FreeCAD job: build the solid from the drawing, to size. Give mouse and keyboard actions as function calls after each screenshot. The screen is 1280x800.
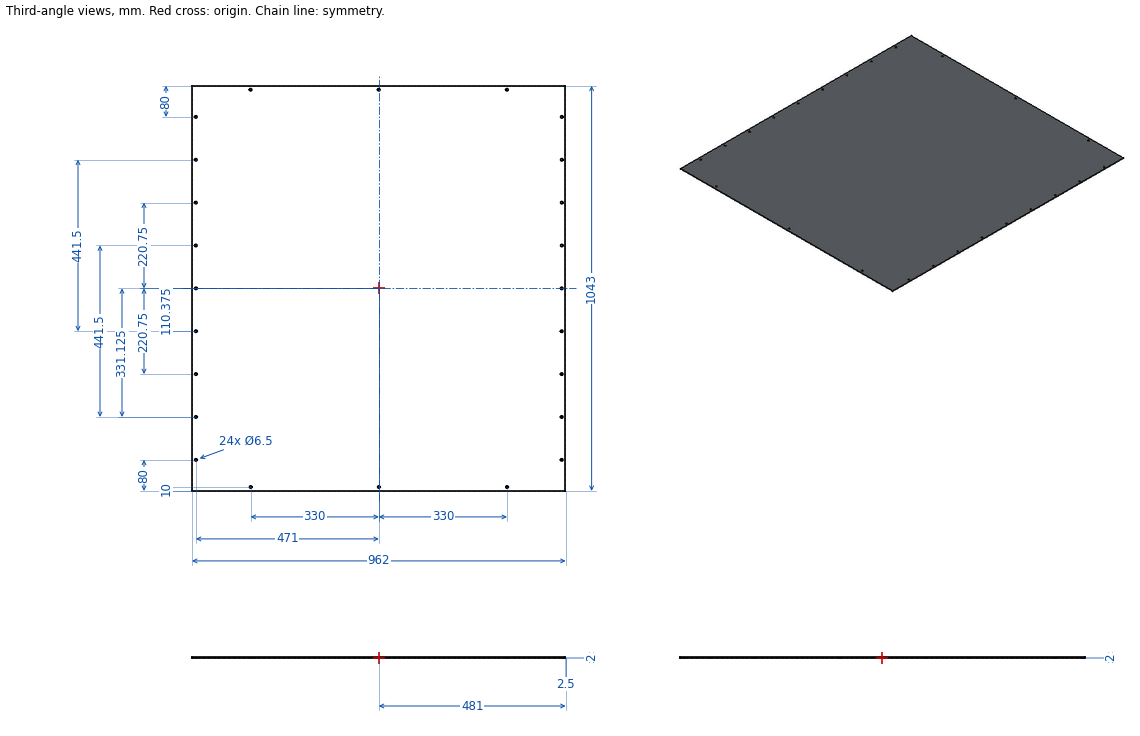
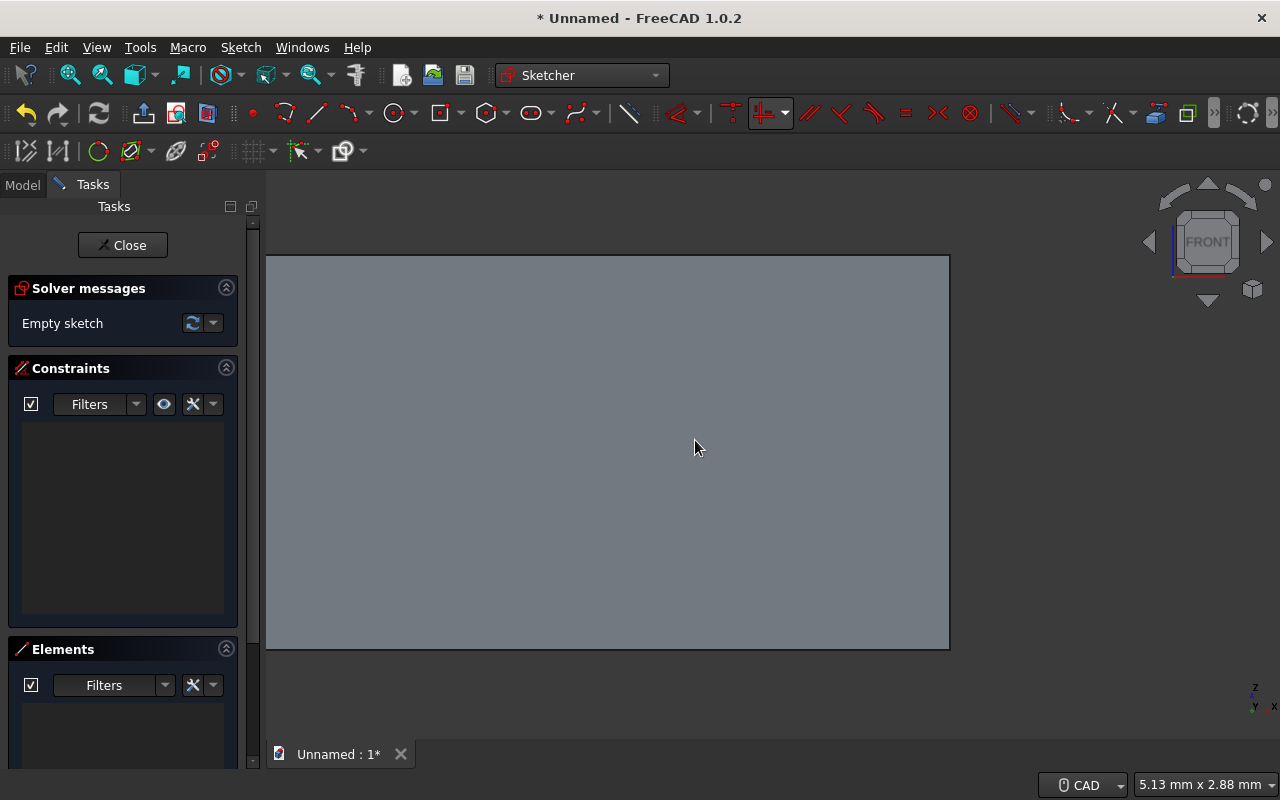
key(g)
key(r)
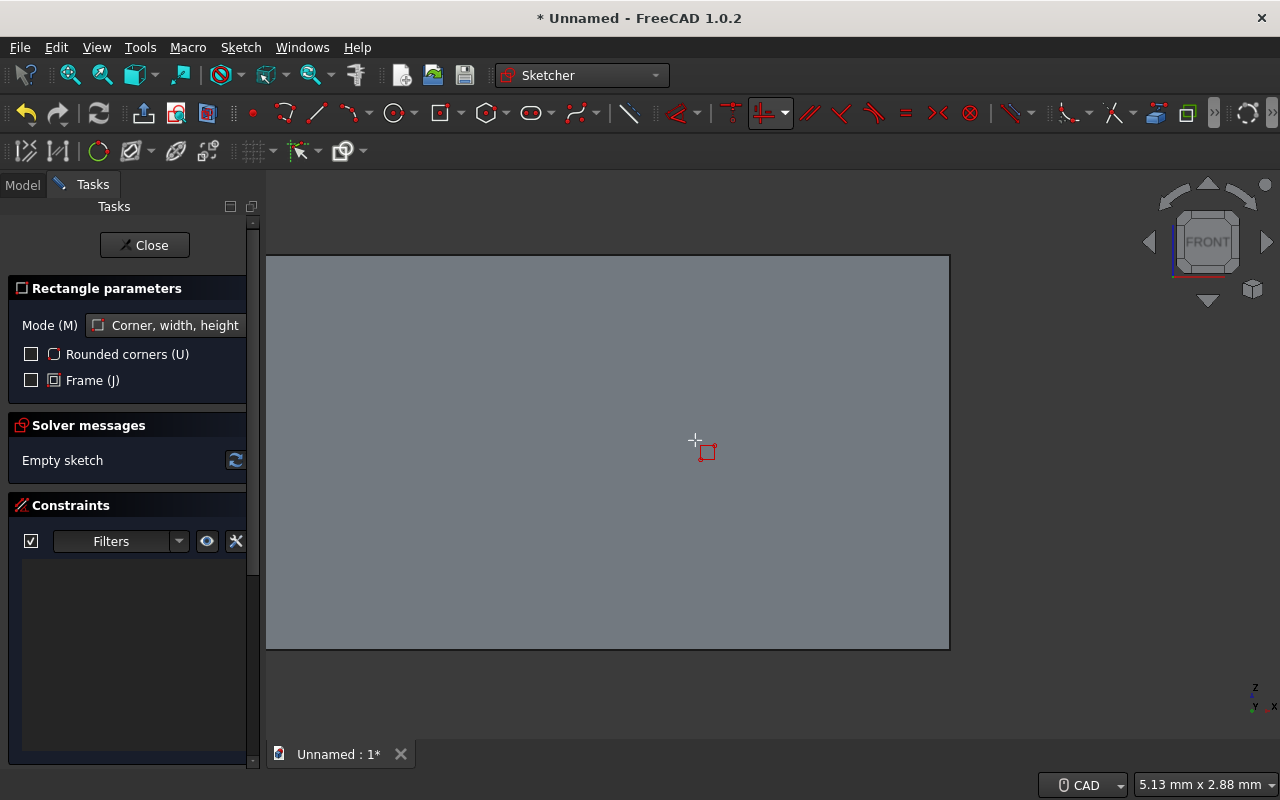
click(456, 255)
click(950, 650)
key(Escape)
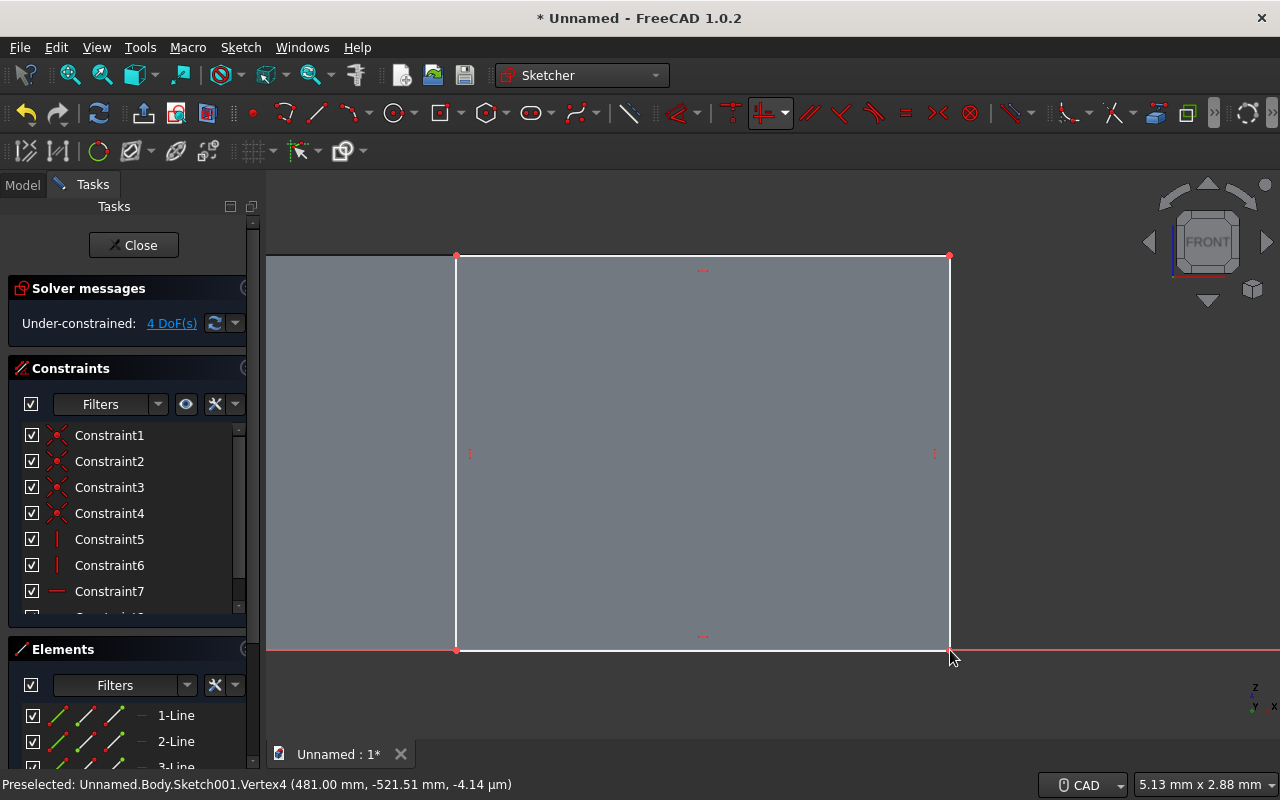
click(456, 651)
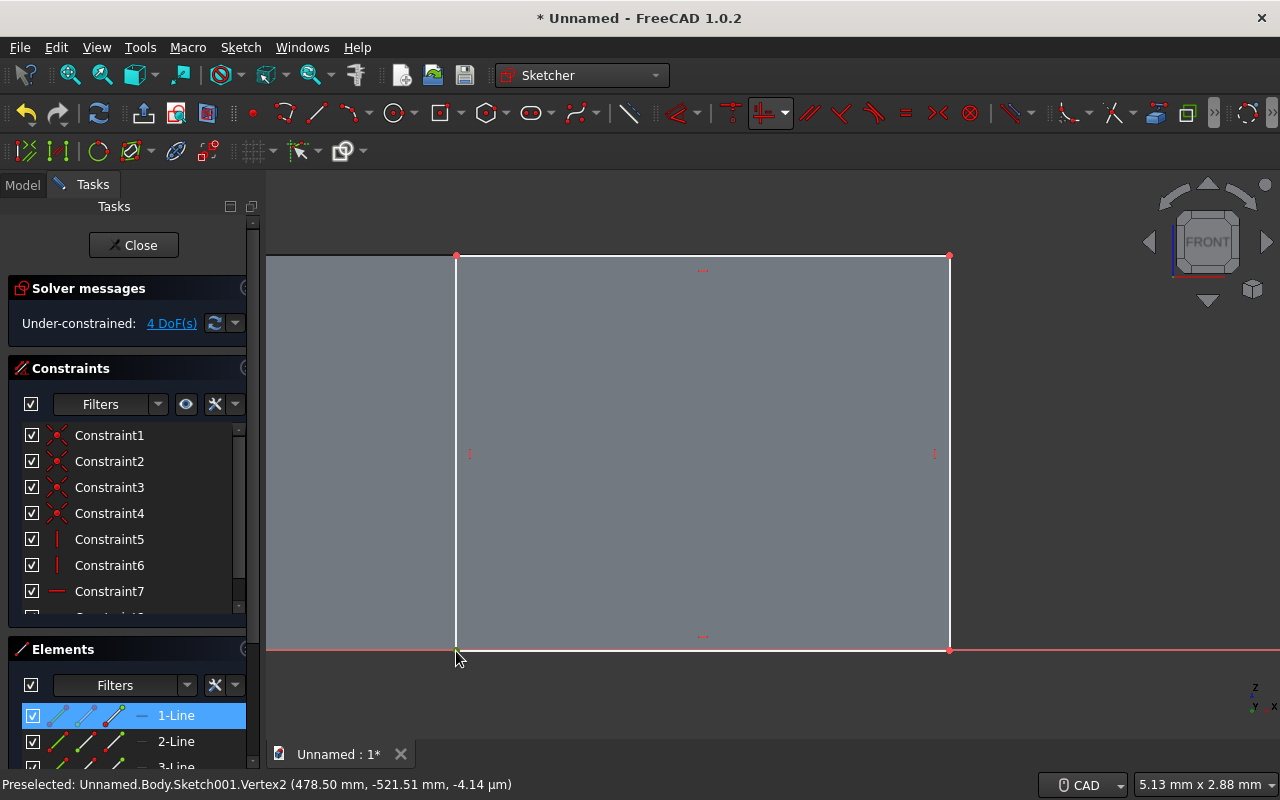
click(353, 650)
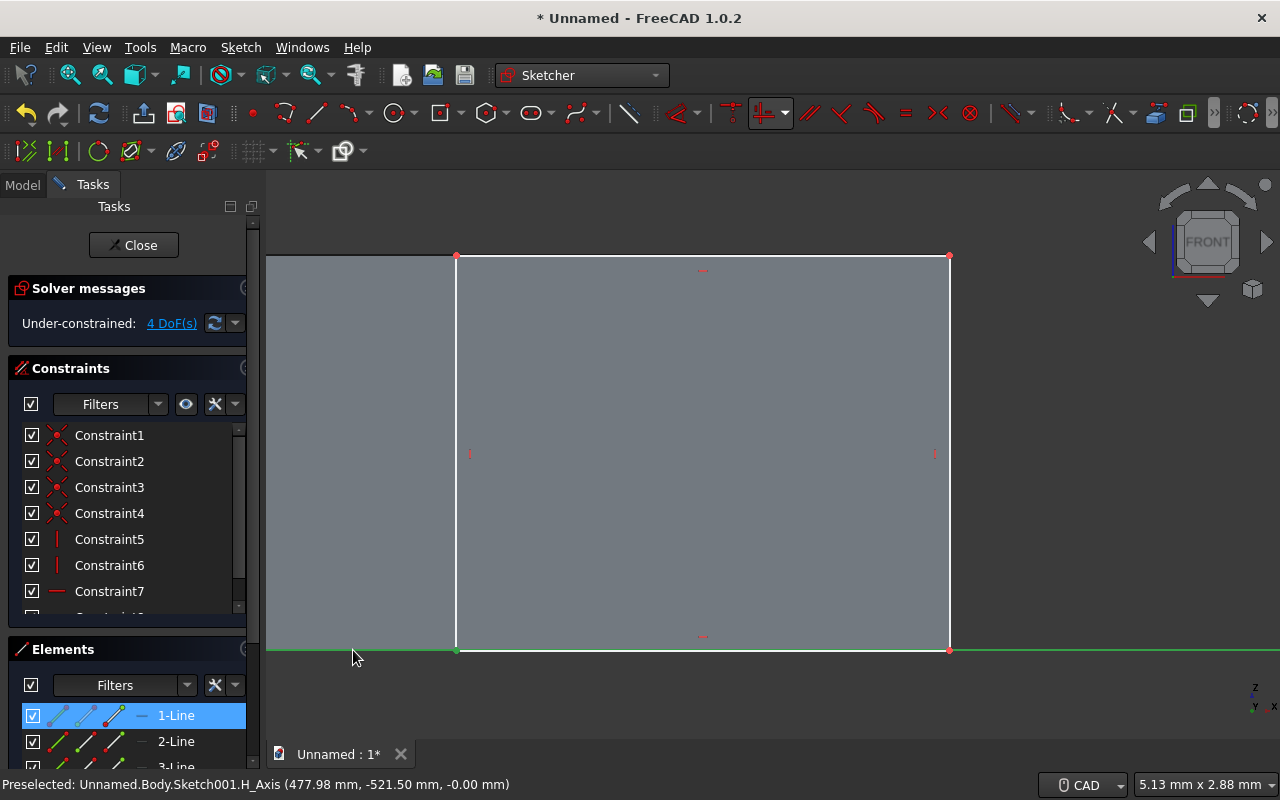
click(732, 114)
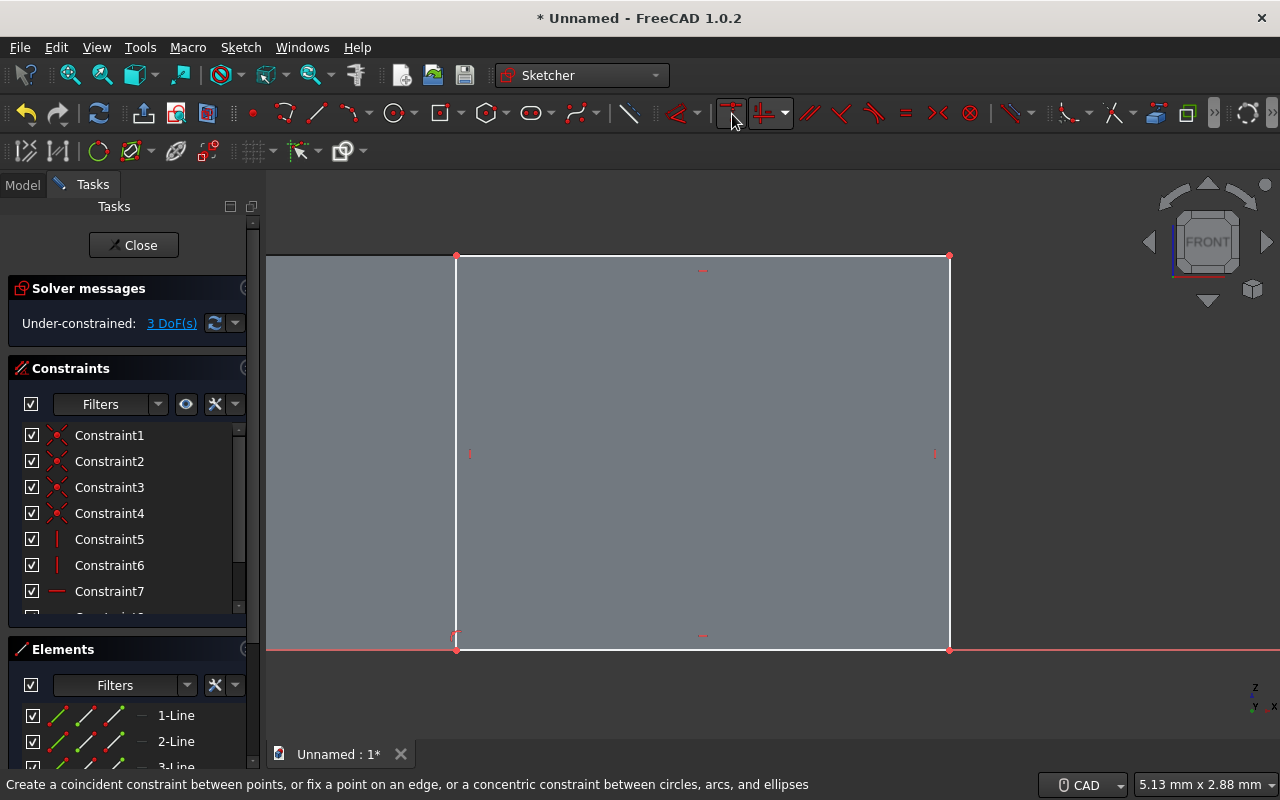
click(676, 114)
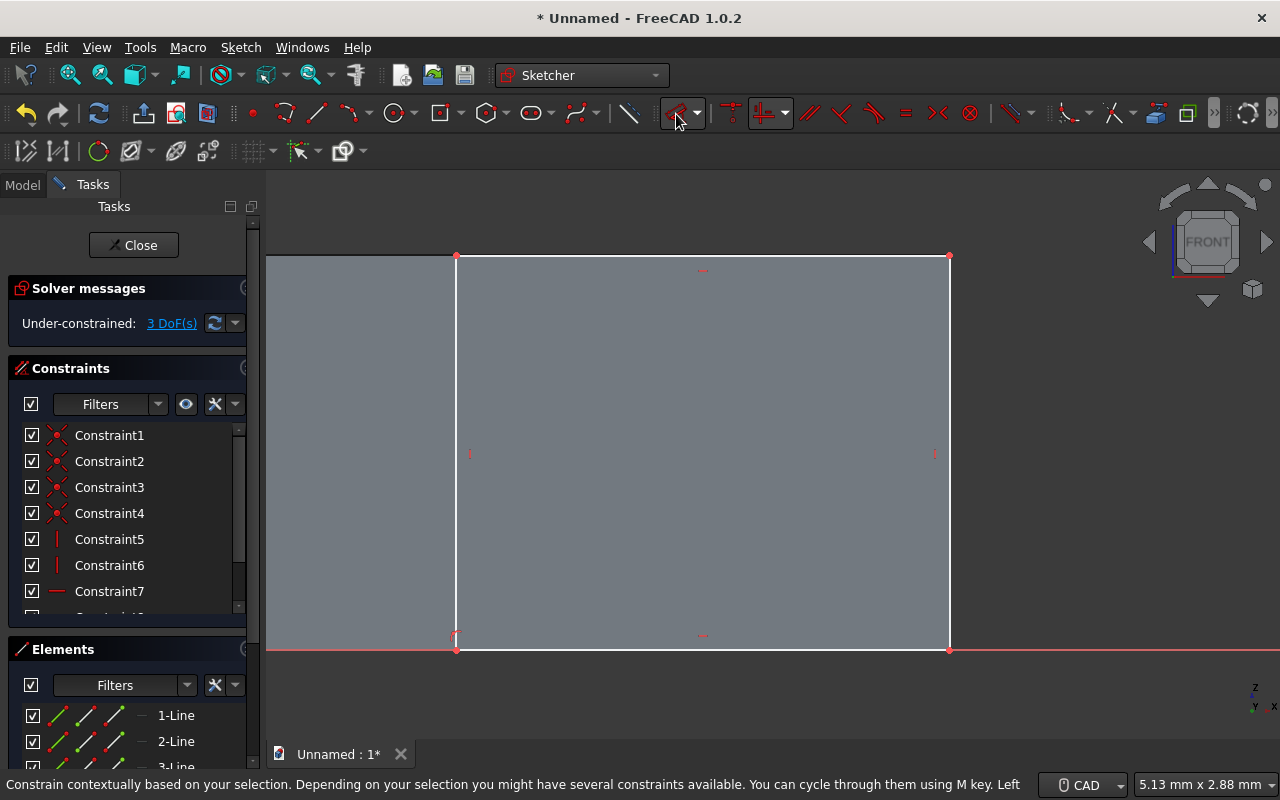
click(456, 374)
click(422, 453)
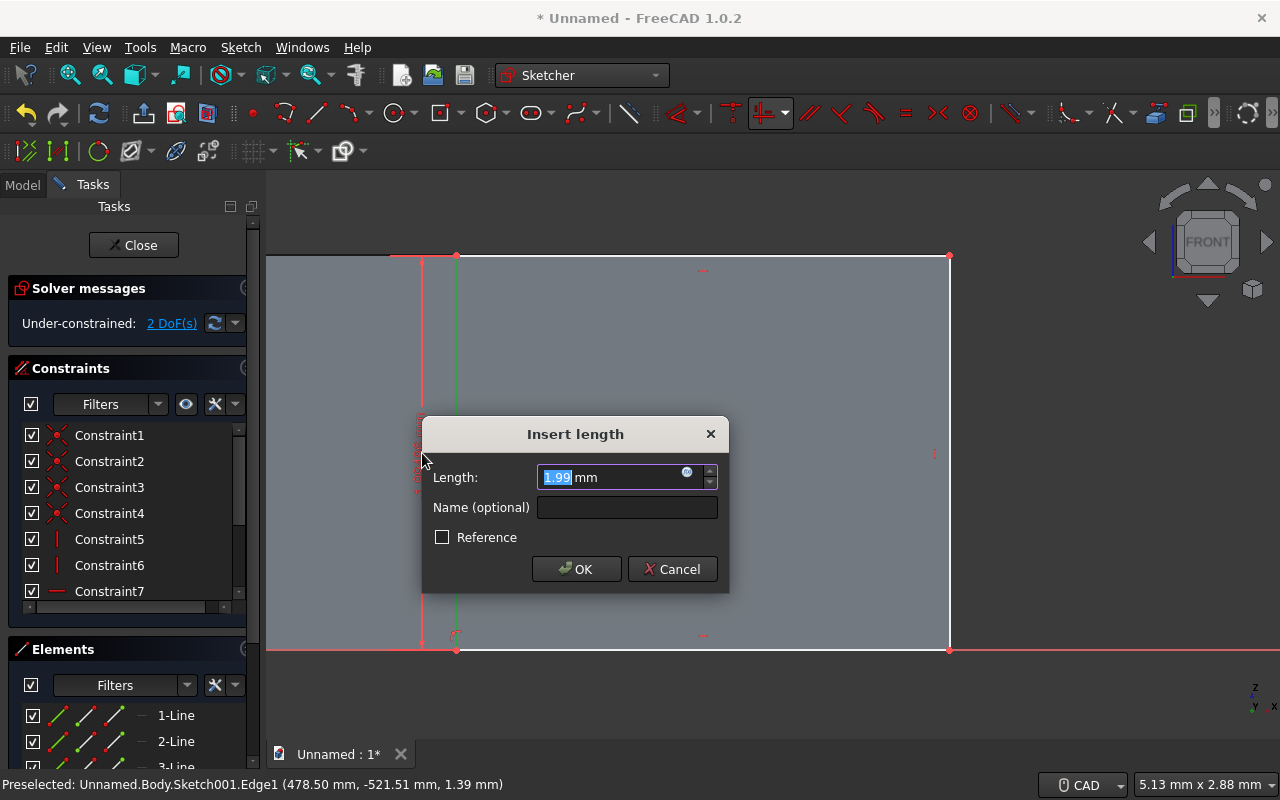
text(2)
key(Return)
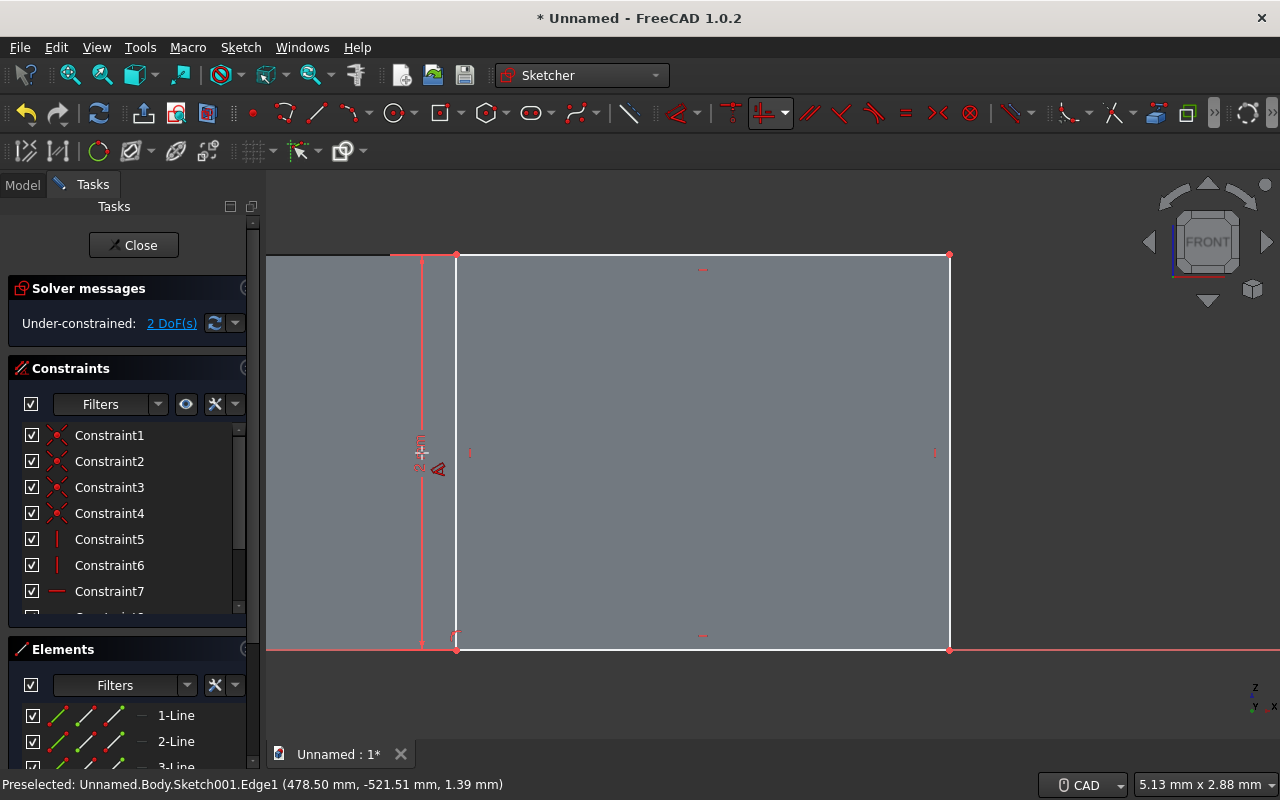
click(604, 650)
click(703, 684)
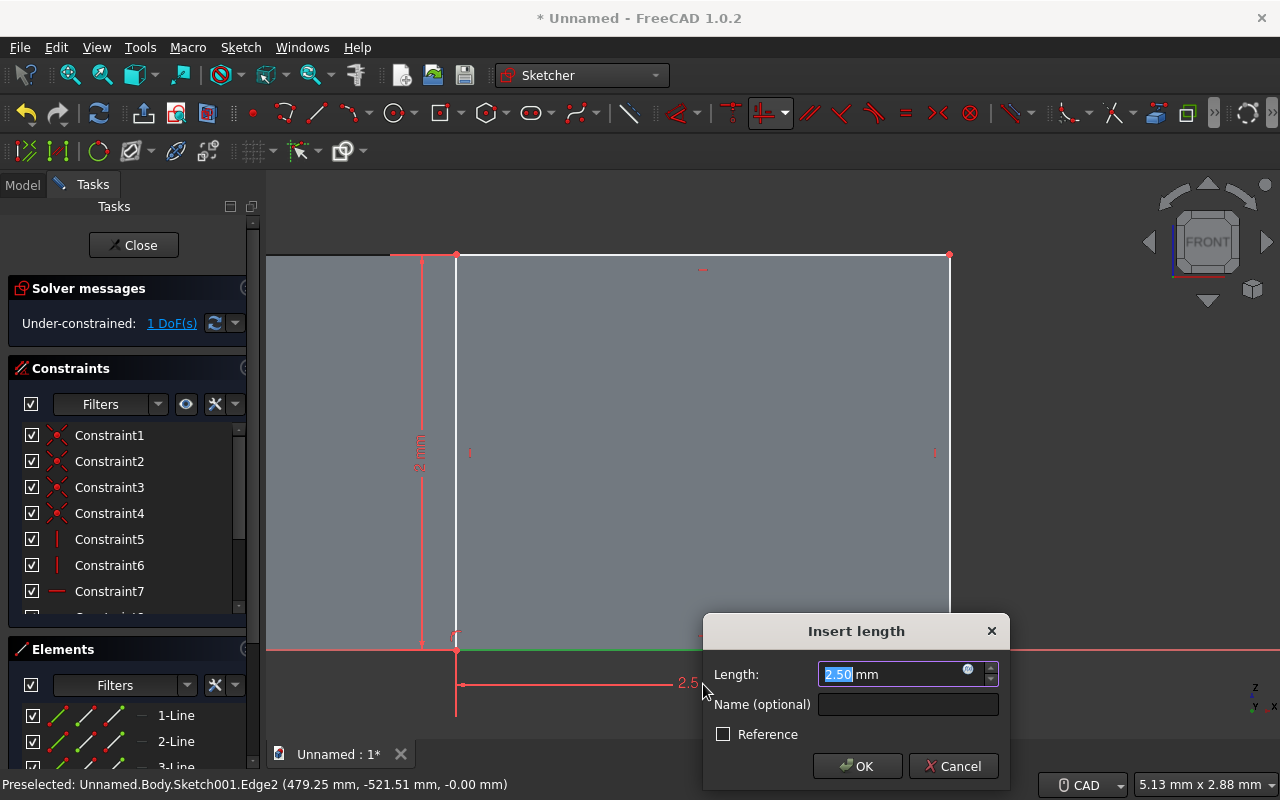
text(2.5)
key(Return)